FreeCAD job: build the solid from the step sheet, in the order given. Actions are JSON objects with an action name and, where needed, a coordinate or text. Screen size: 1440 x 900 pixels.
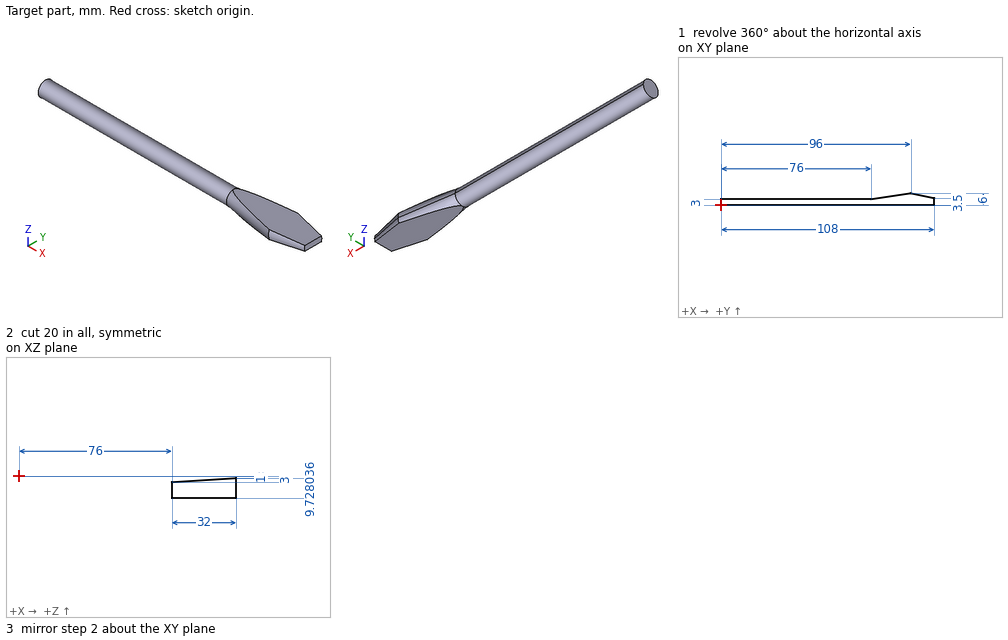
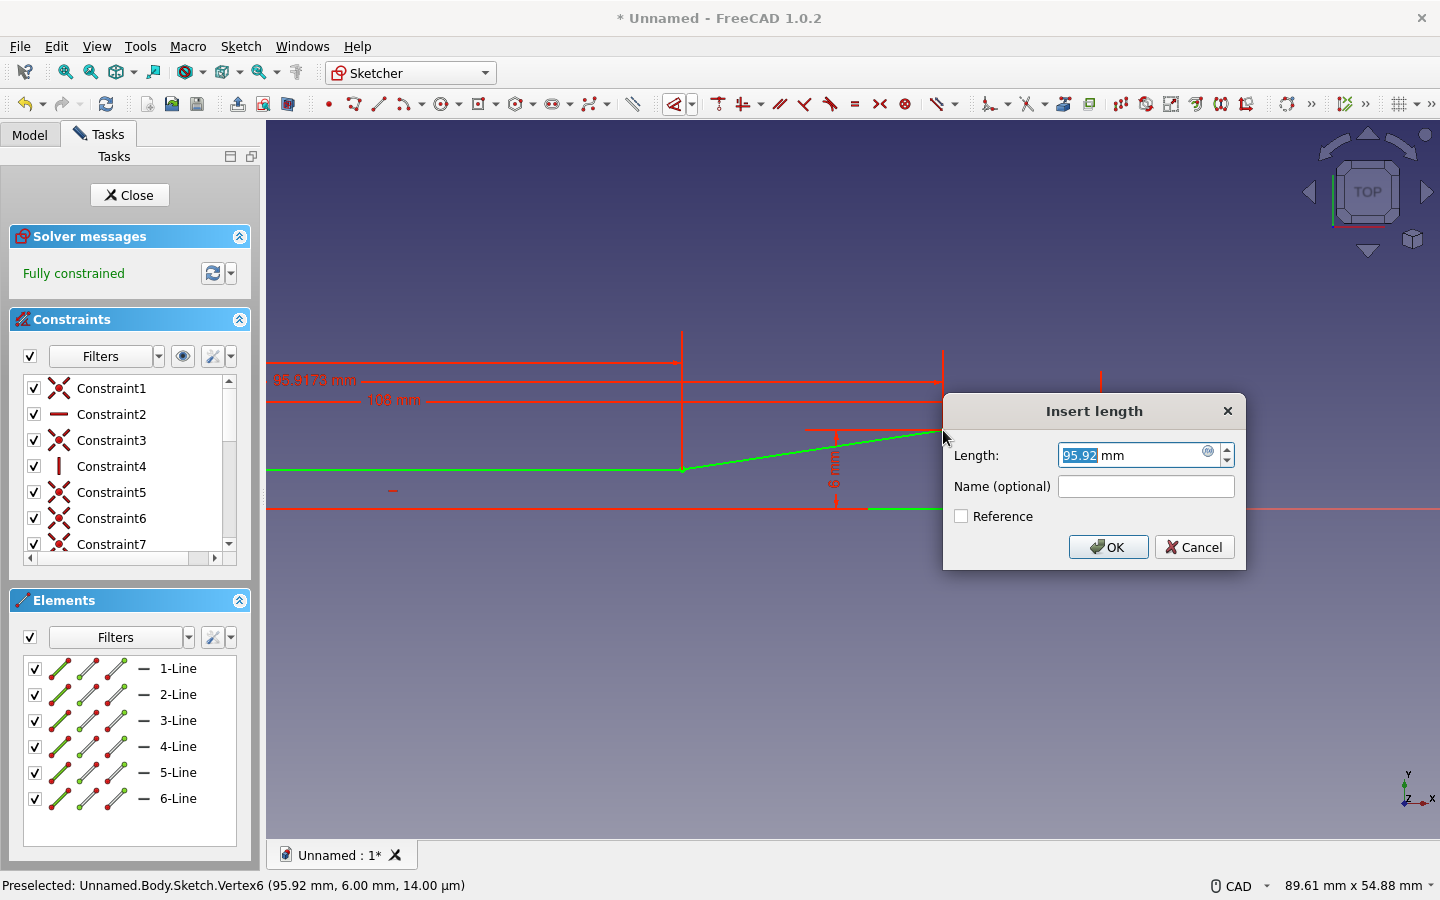
{"action": "type", "text": "96"}
{"action": "key", "text": "Return"}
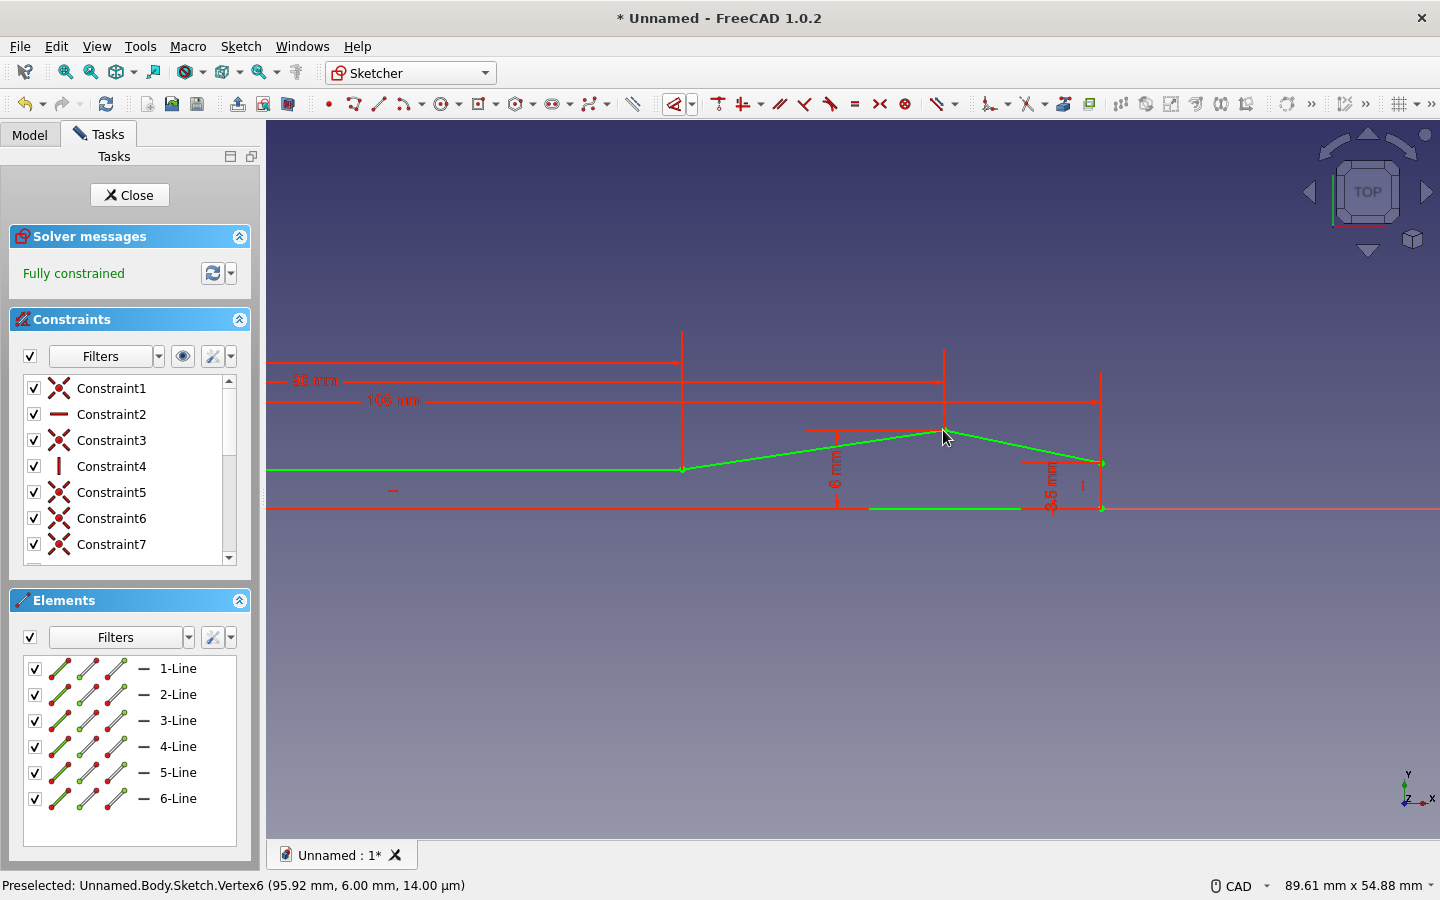
{"action": "left_click", "coordinate": [130, 195]}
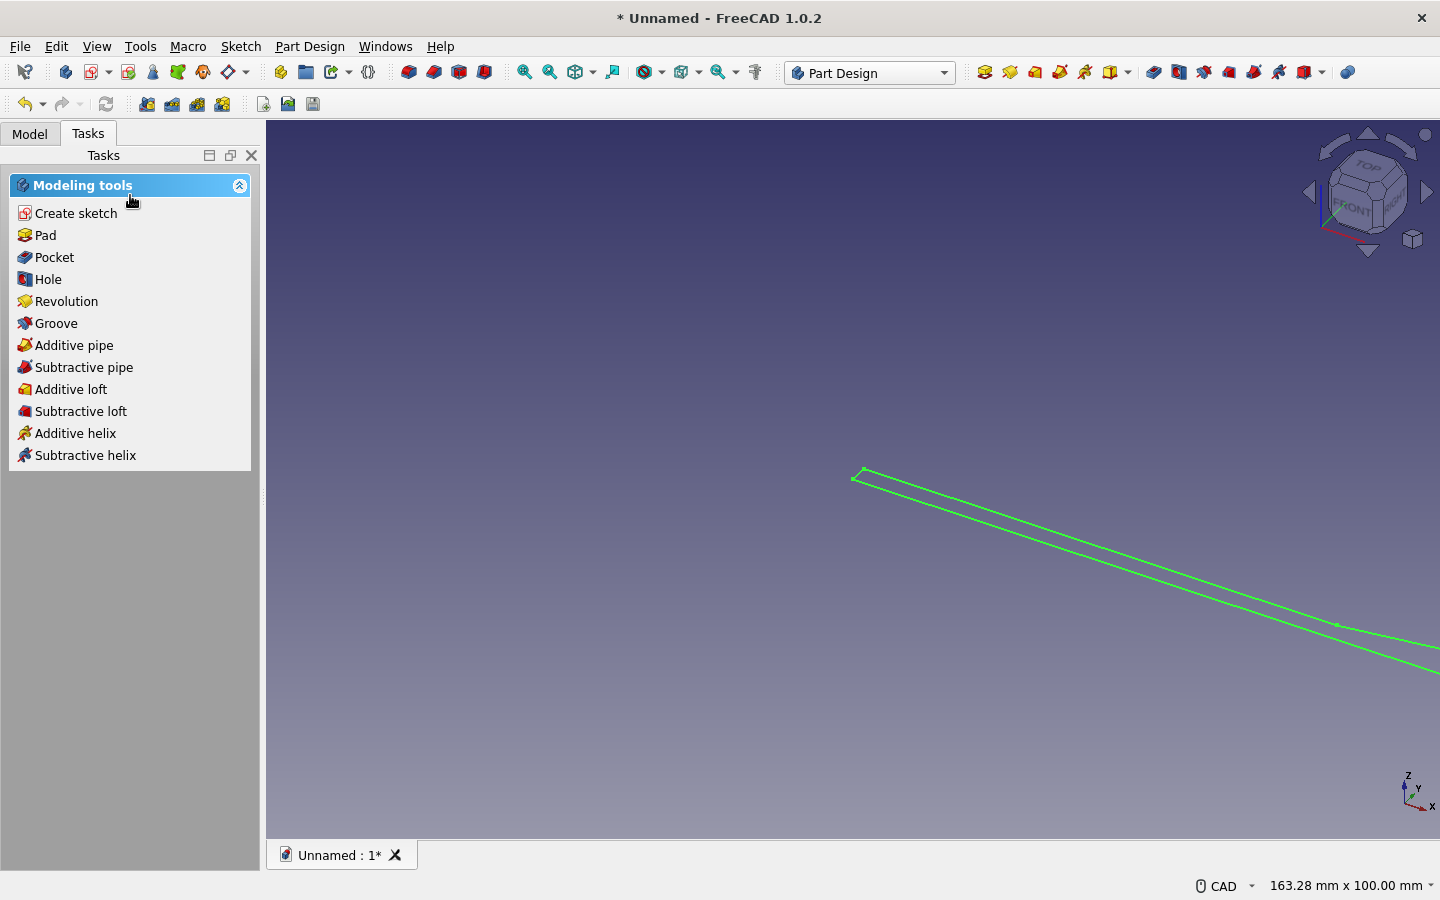
{"action": "left_click", "coordinate": [1010, 72]}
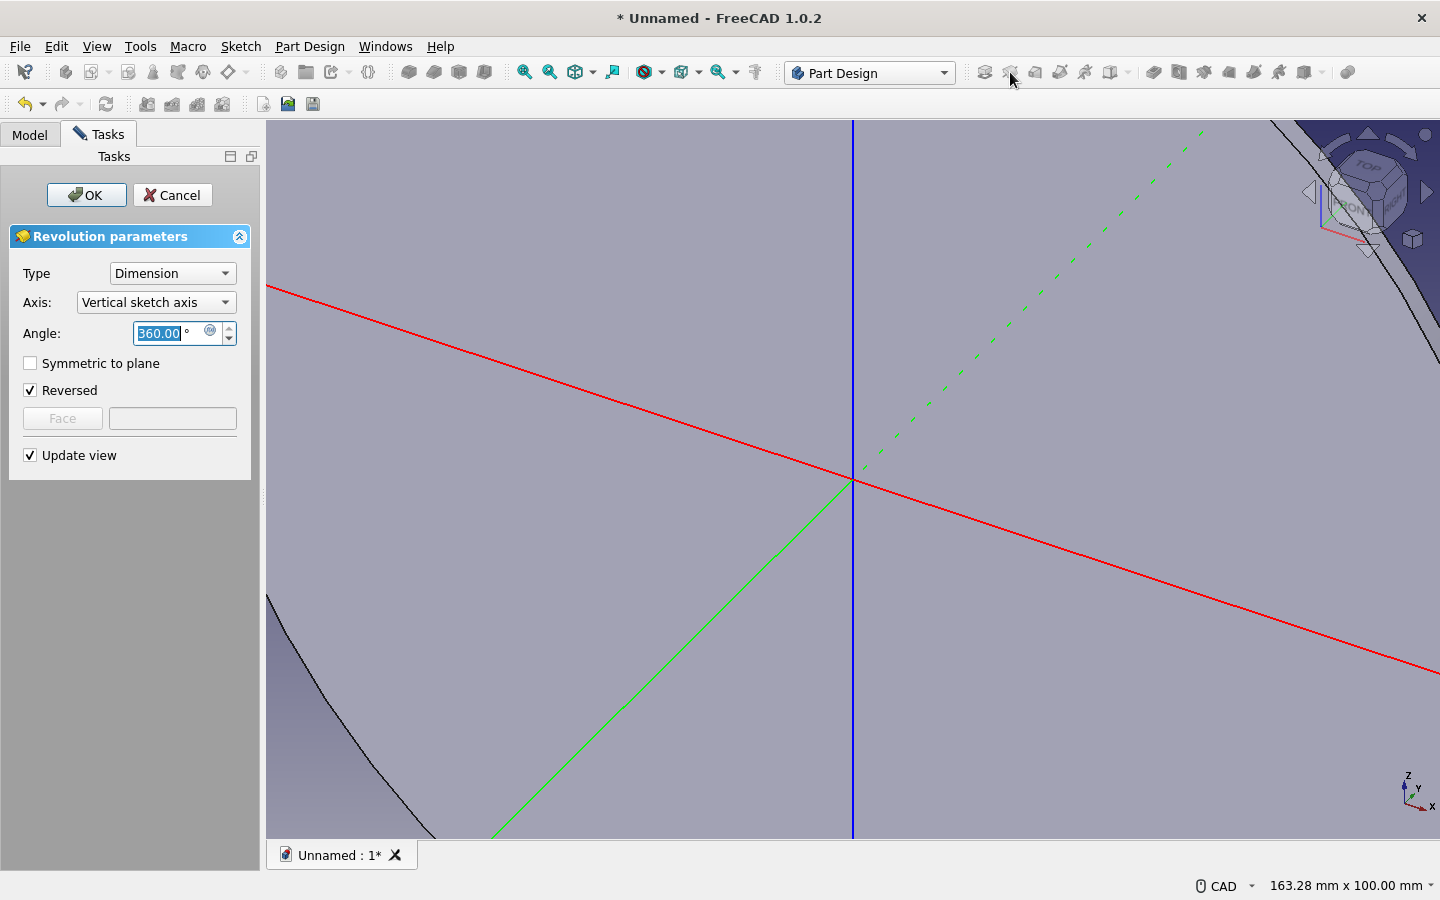
{"action": "left_click", "coordinate": [157, 302]}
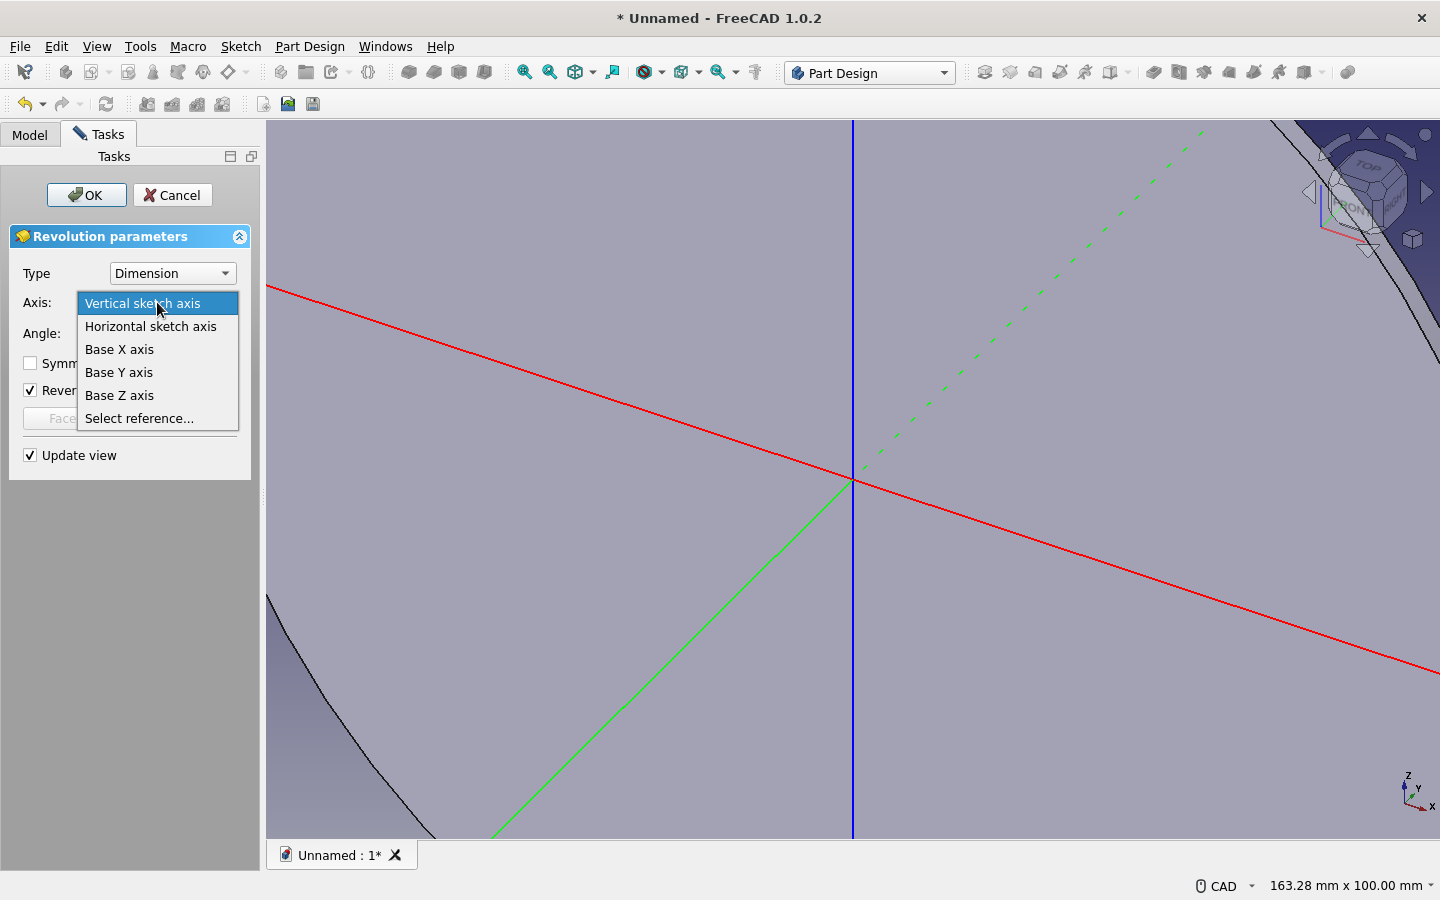
{"action": "left_click", "coordinate": [156, 326]}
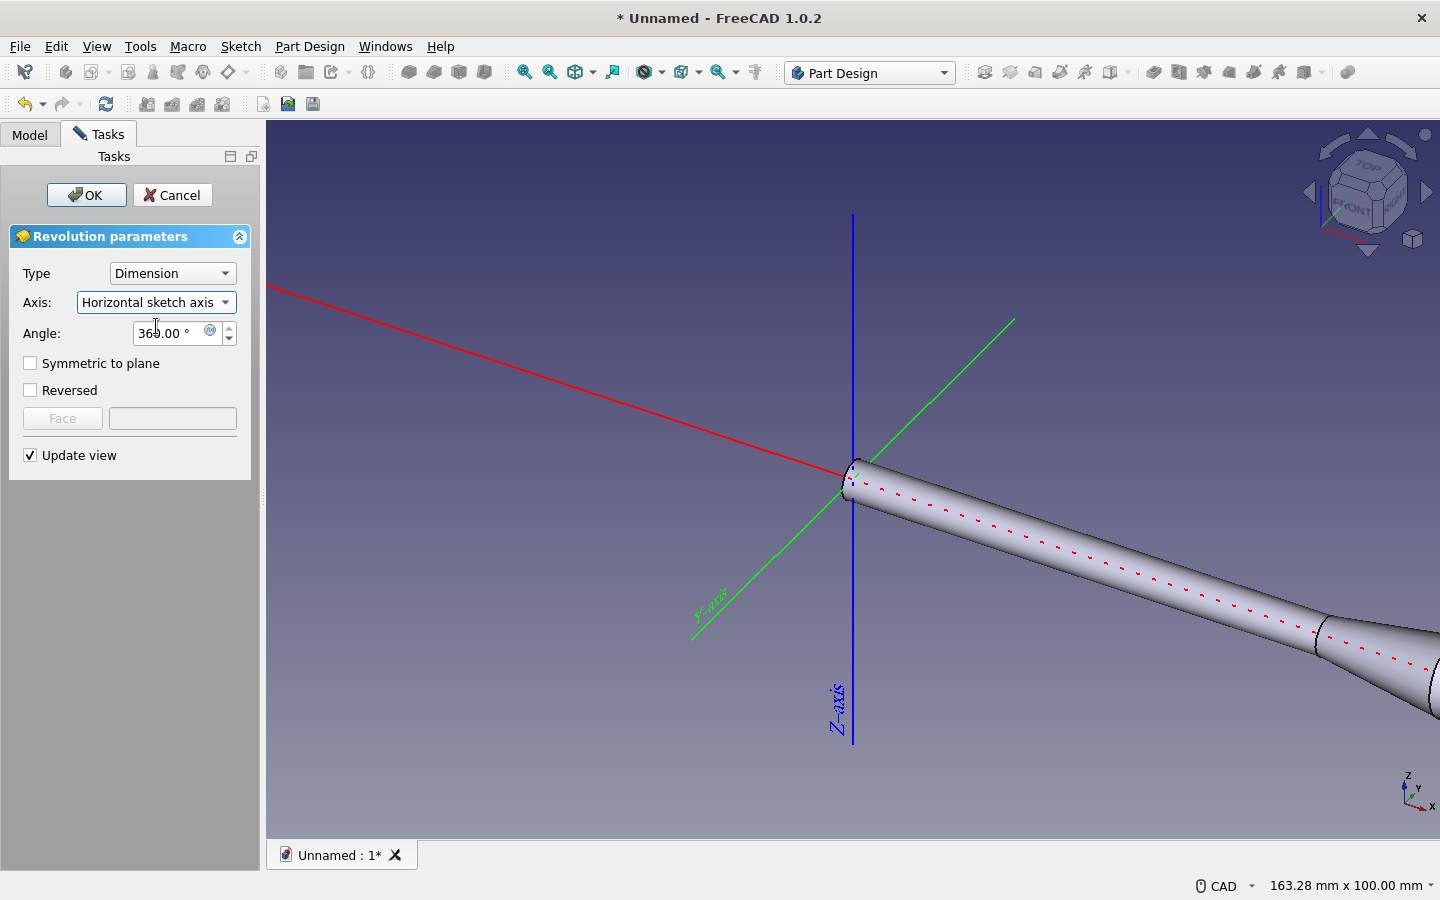
{"action": "left_click", "coordinate": [87, 195]}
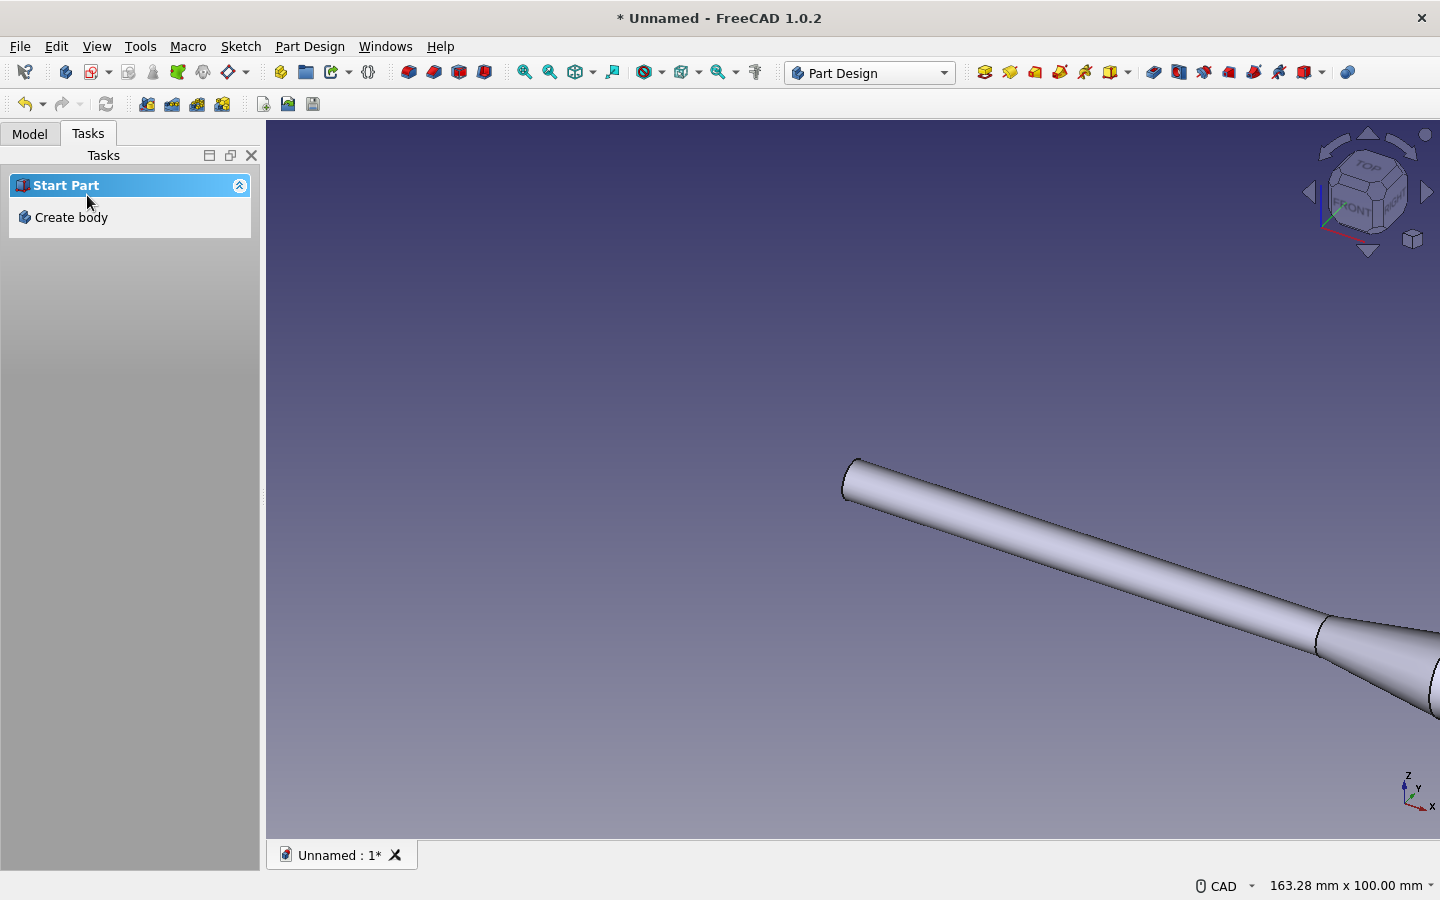
{"action": "left_click", "coordinate": [525, 72]}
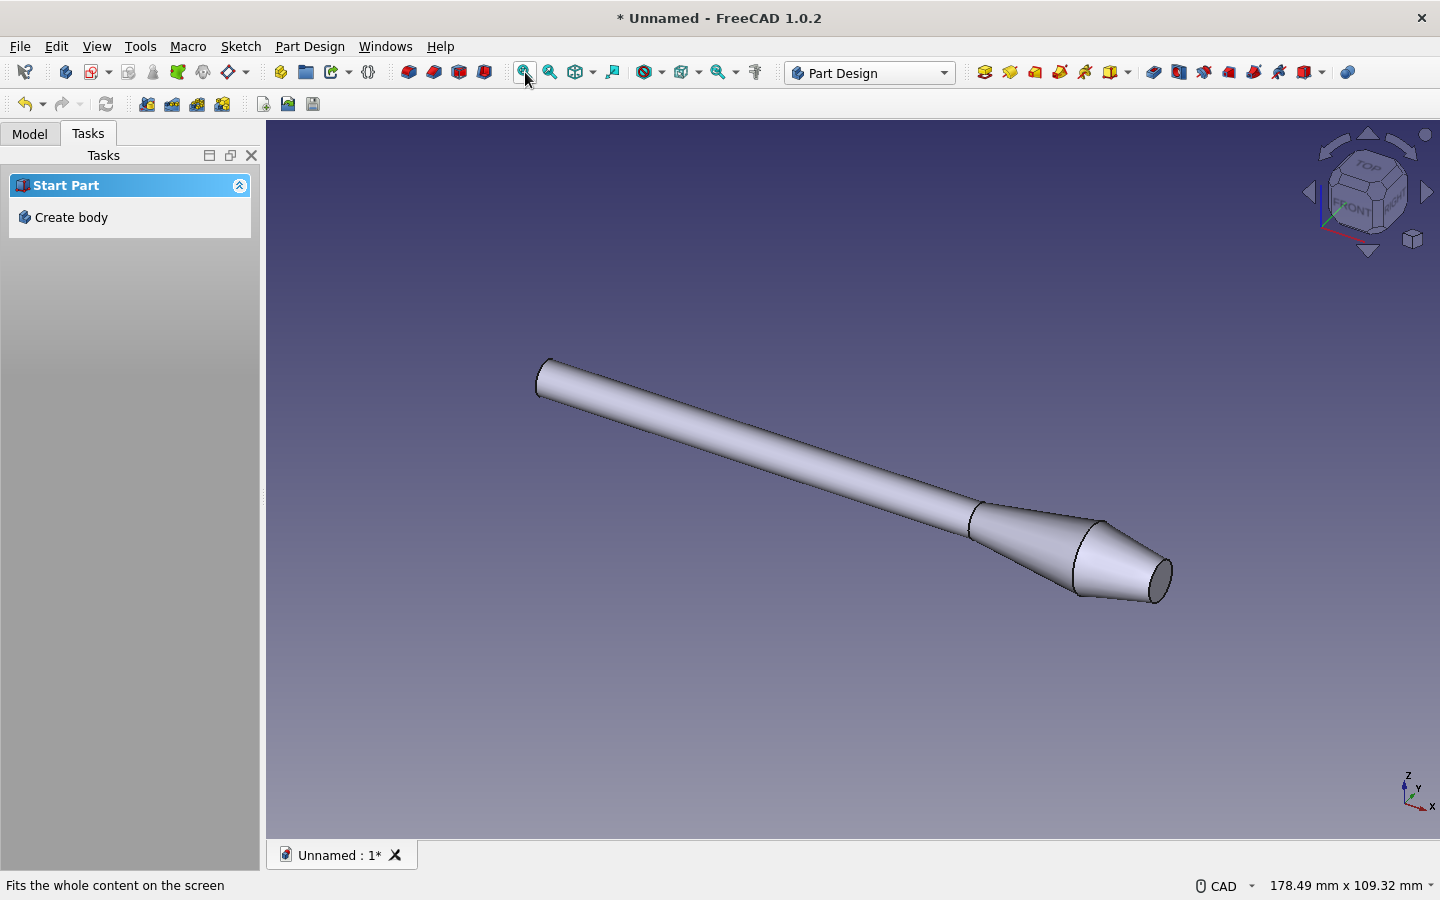
{"action": "left_click", "coordinate": [90, 72]}